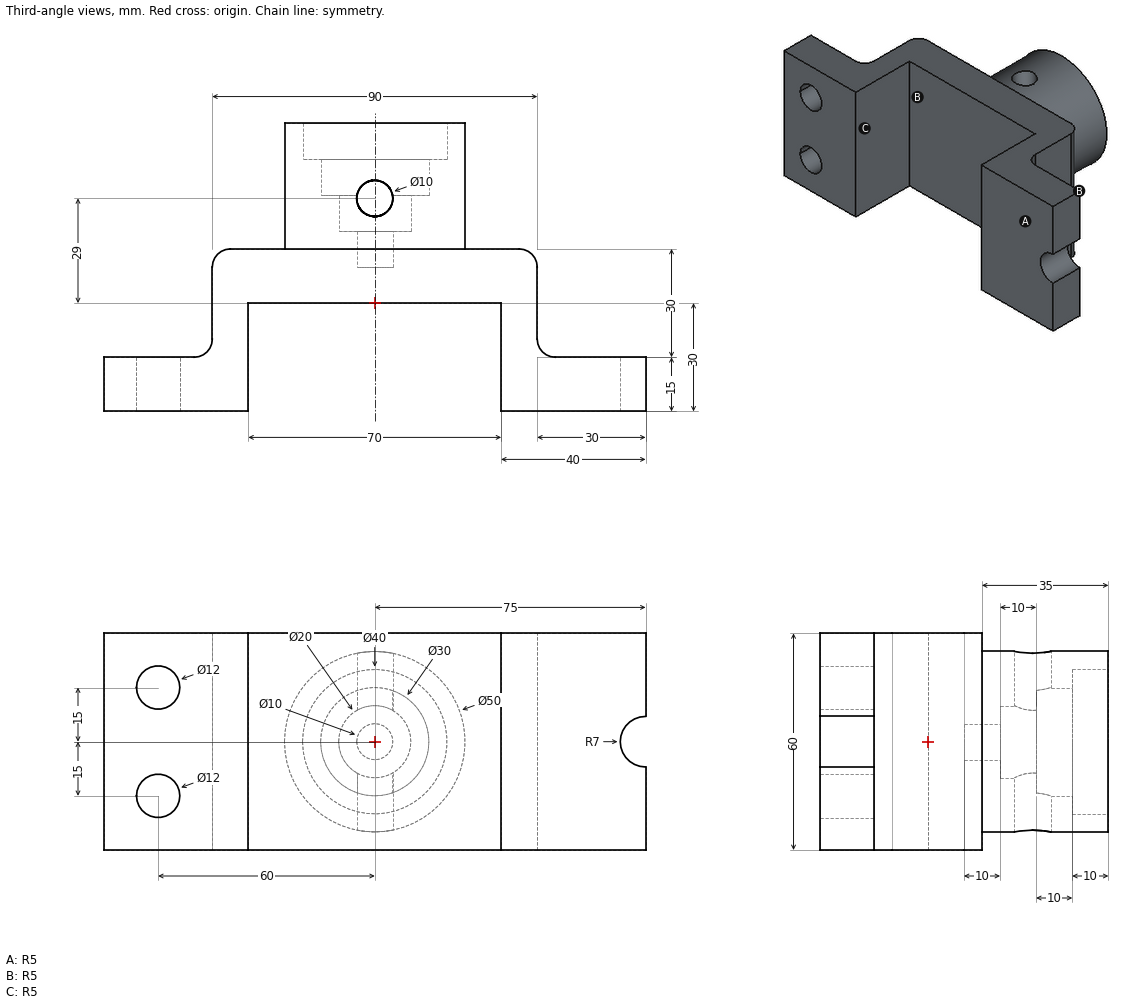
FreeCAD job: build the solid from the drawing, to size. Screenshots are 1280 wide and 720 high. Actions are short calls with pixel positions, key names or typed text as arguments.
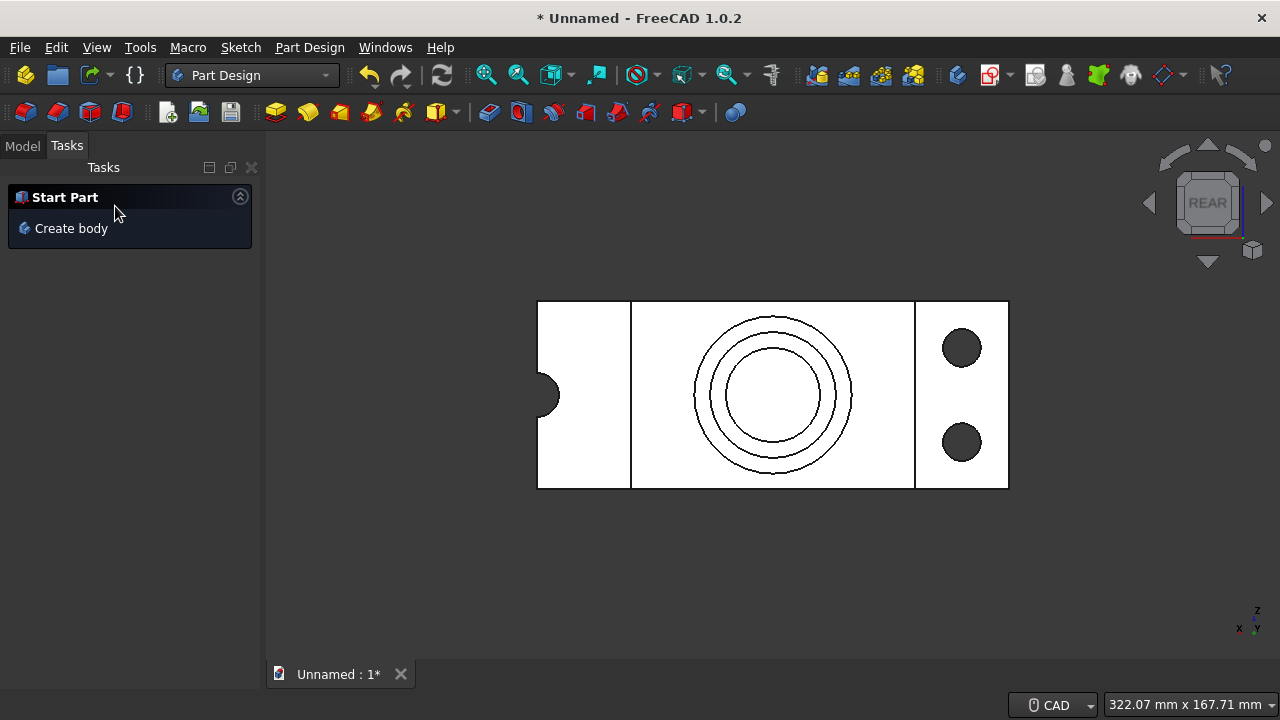
click(773, 394)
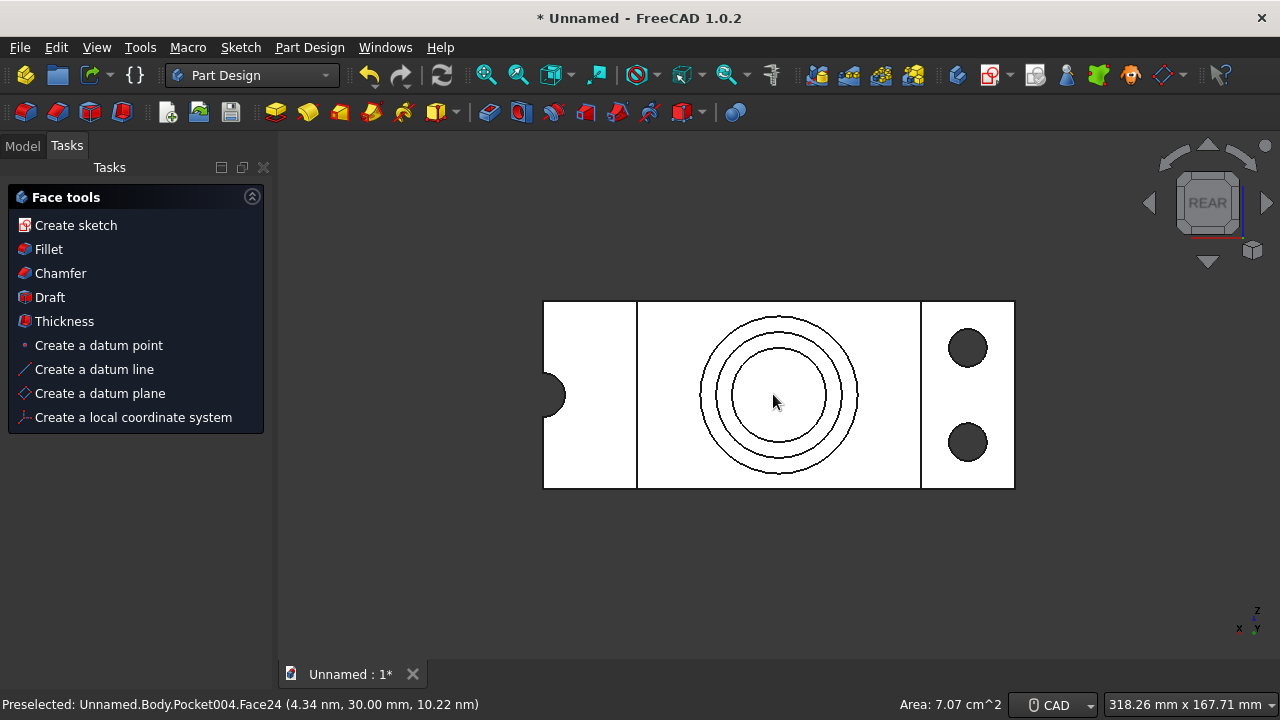
click(990, 76)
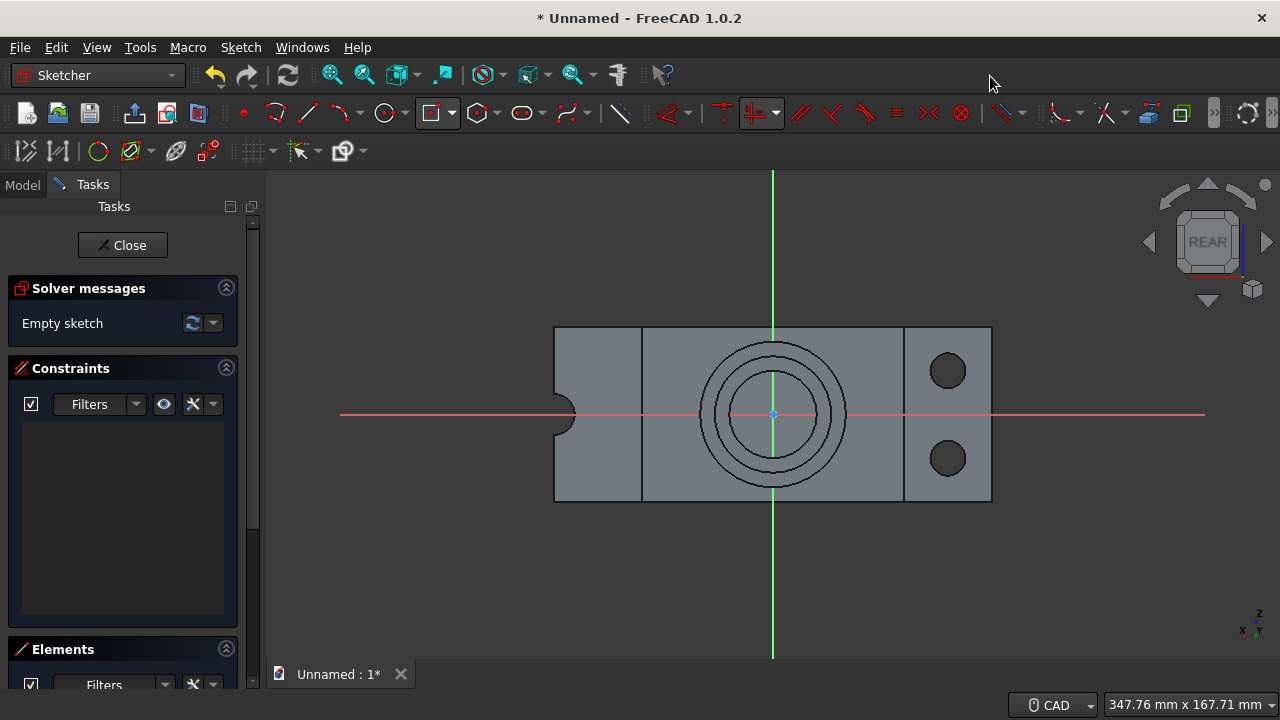
key(q)
key(s)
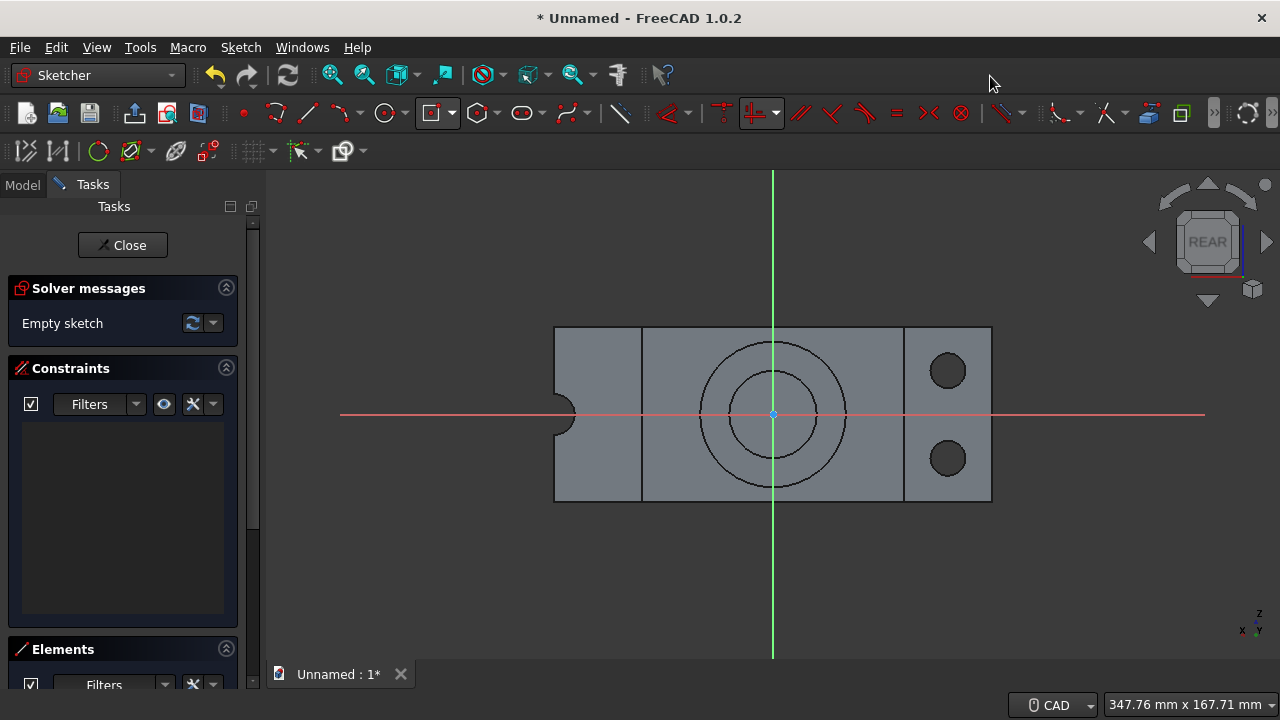
scroll(790, 415, up, 8)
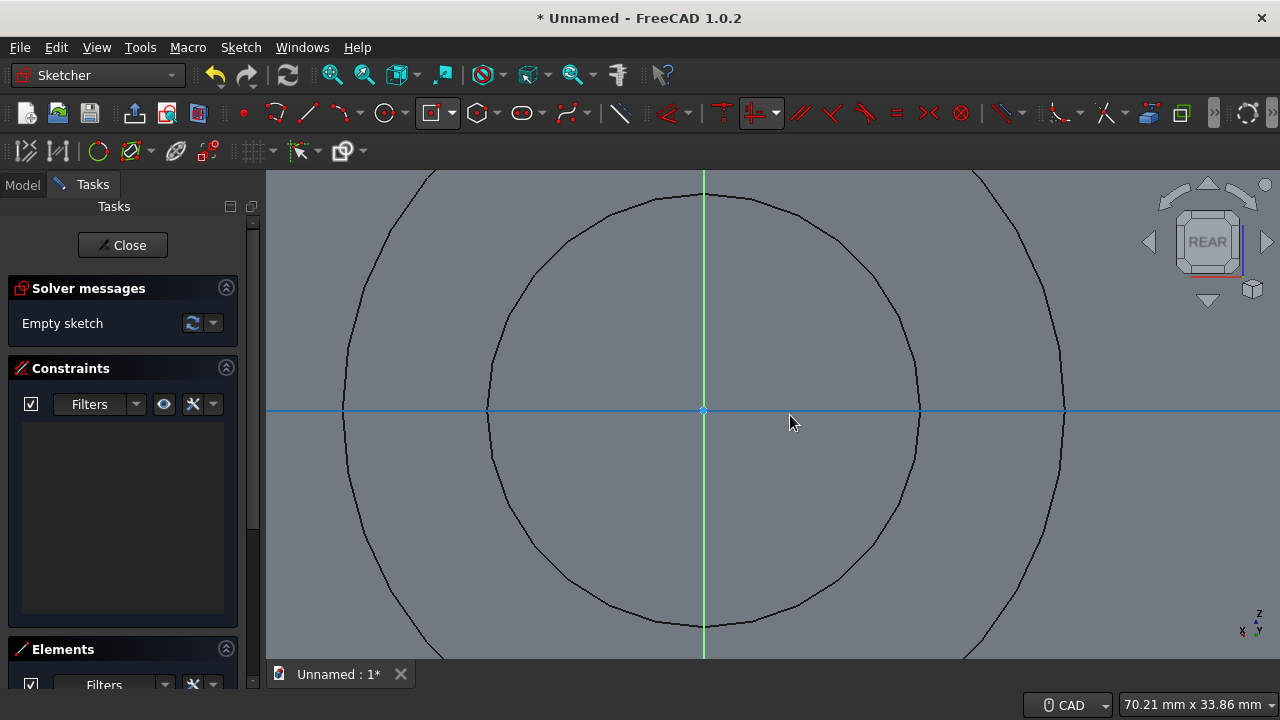
click(386, 114)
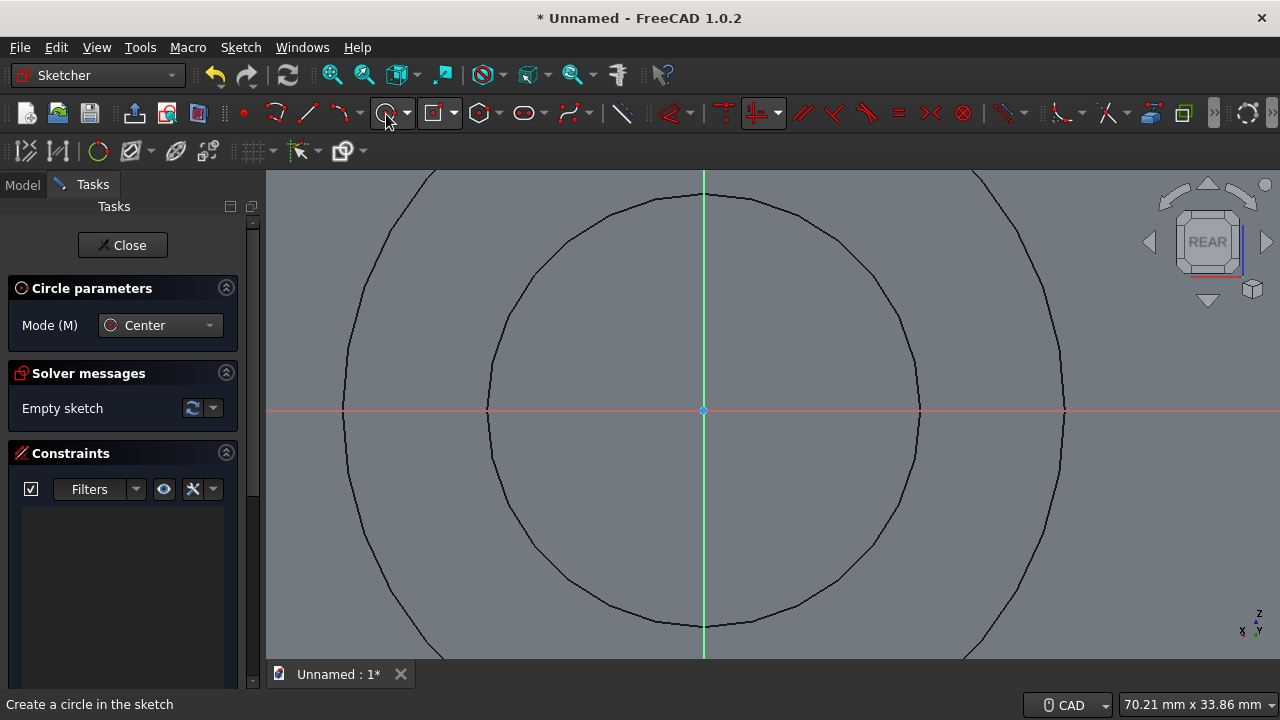
click(704, 411)
click(806, 308)
key(Escape)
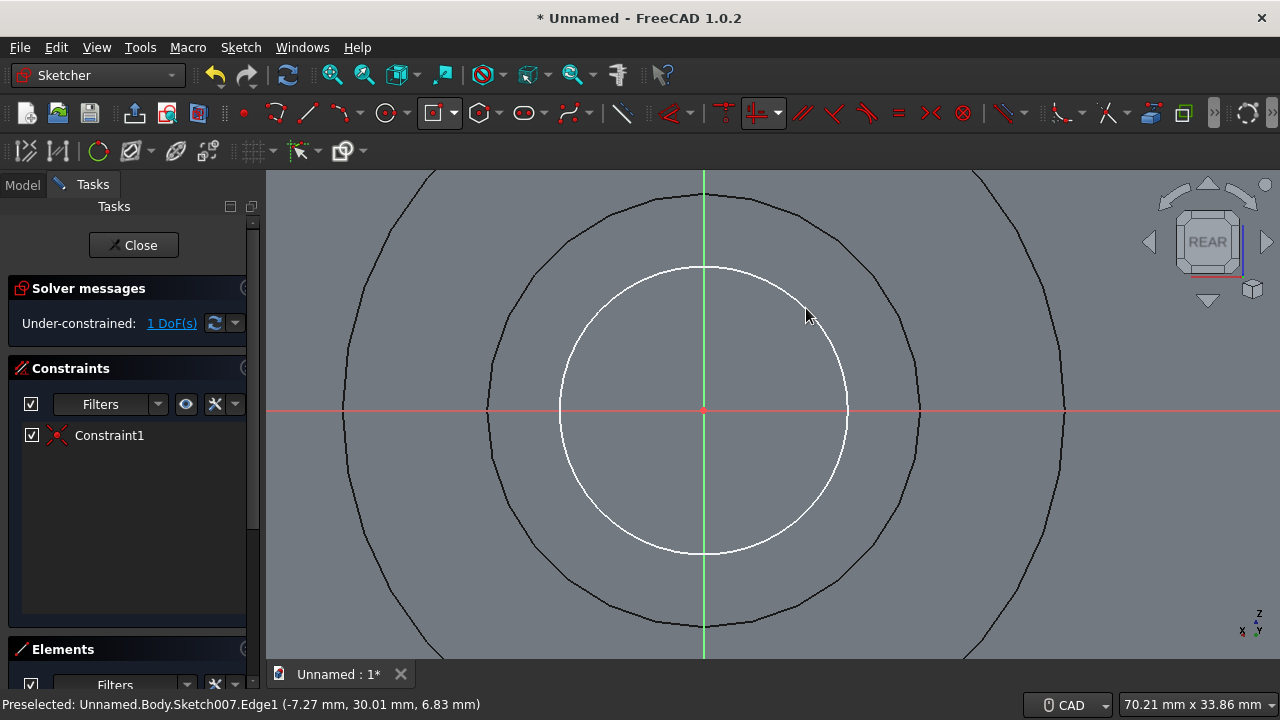
click(670, 114)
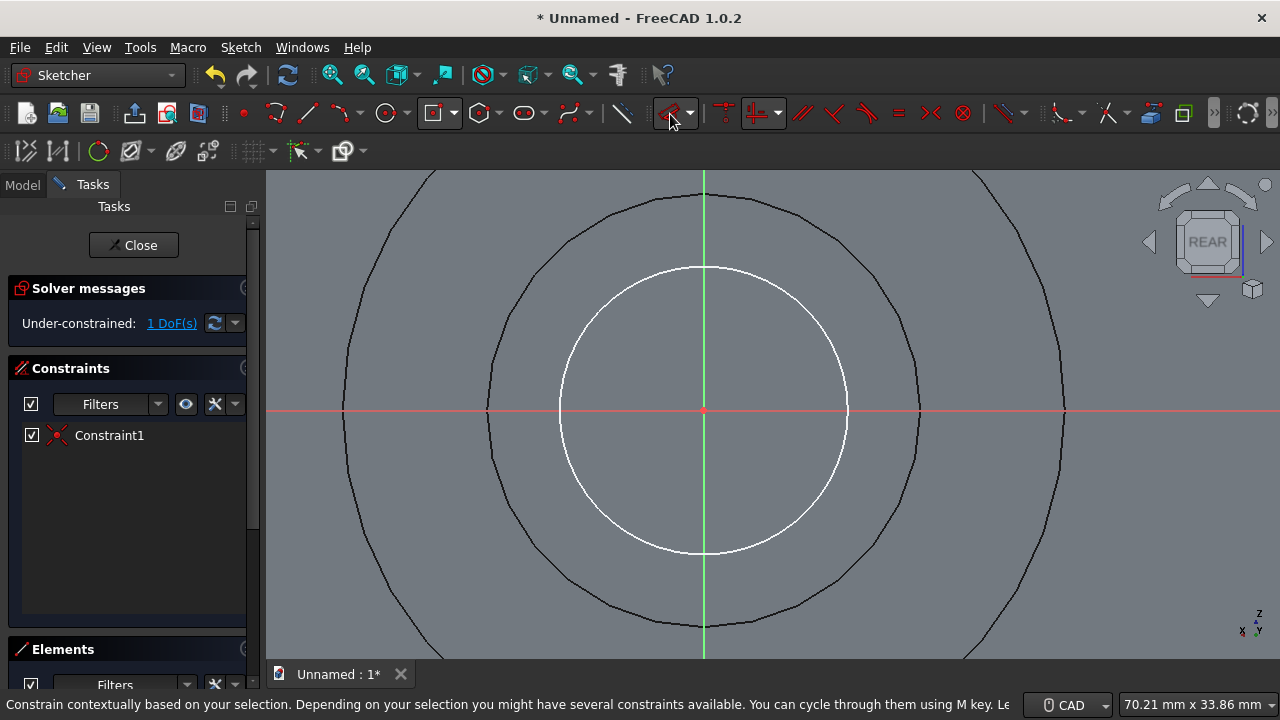
click(805, 308)
click(827, 285)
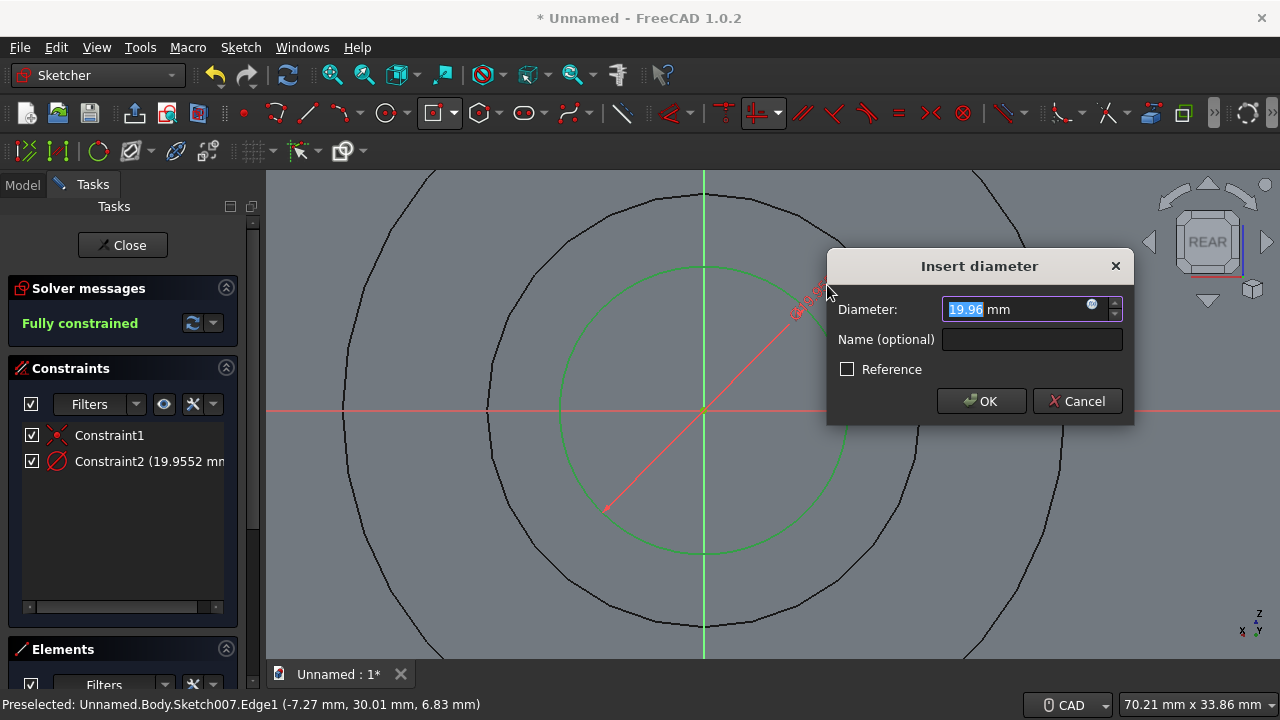
text(20)
key(Return)
key(Escape)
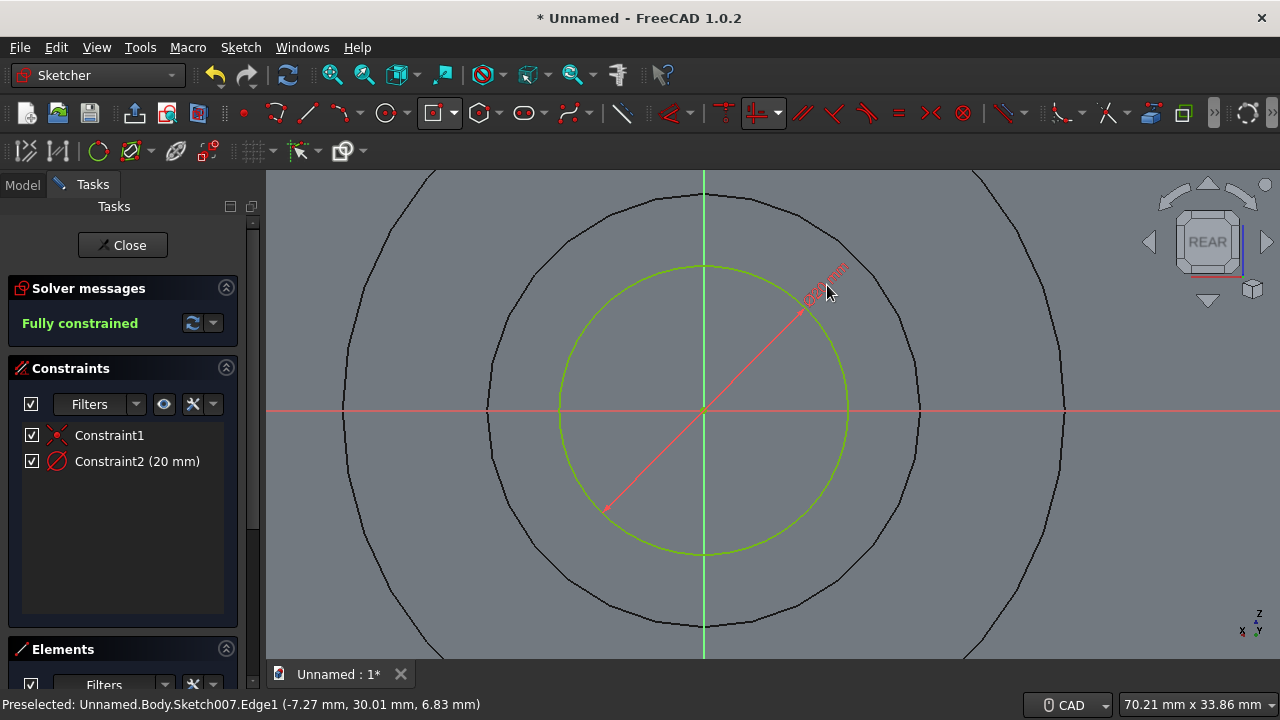
click(123, 245)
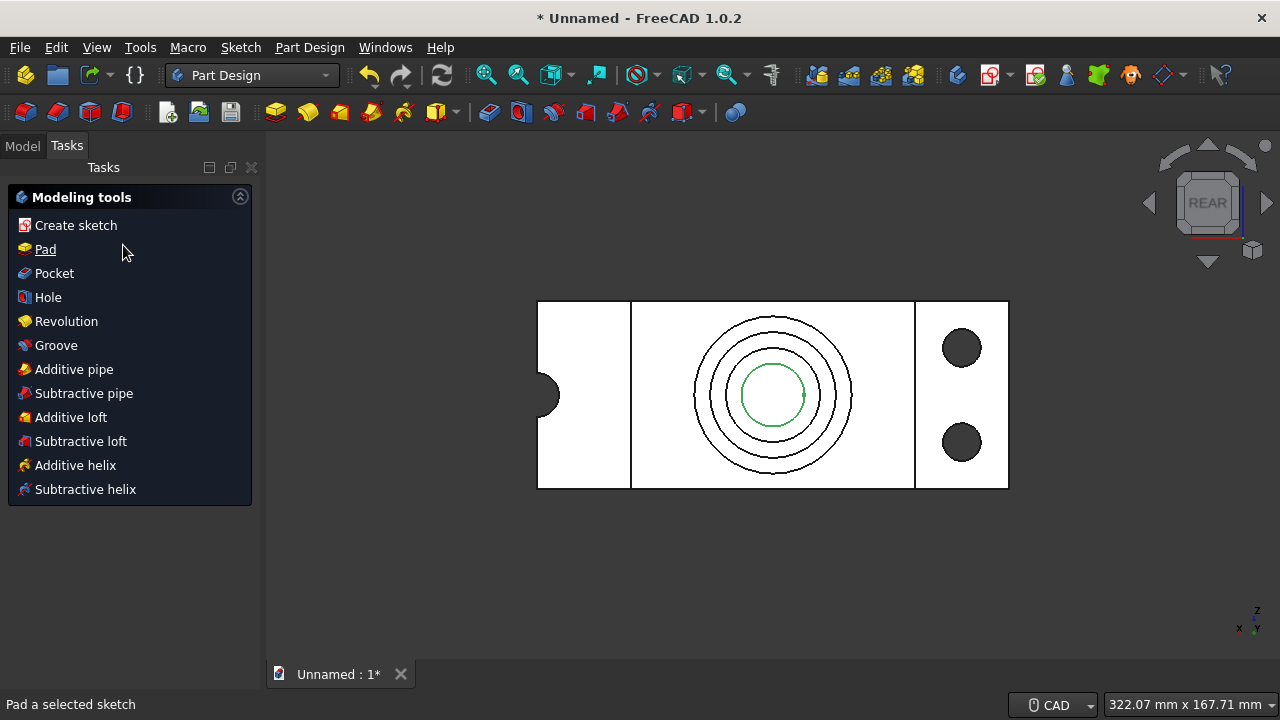
click(490, 112)